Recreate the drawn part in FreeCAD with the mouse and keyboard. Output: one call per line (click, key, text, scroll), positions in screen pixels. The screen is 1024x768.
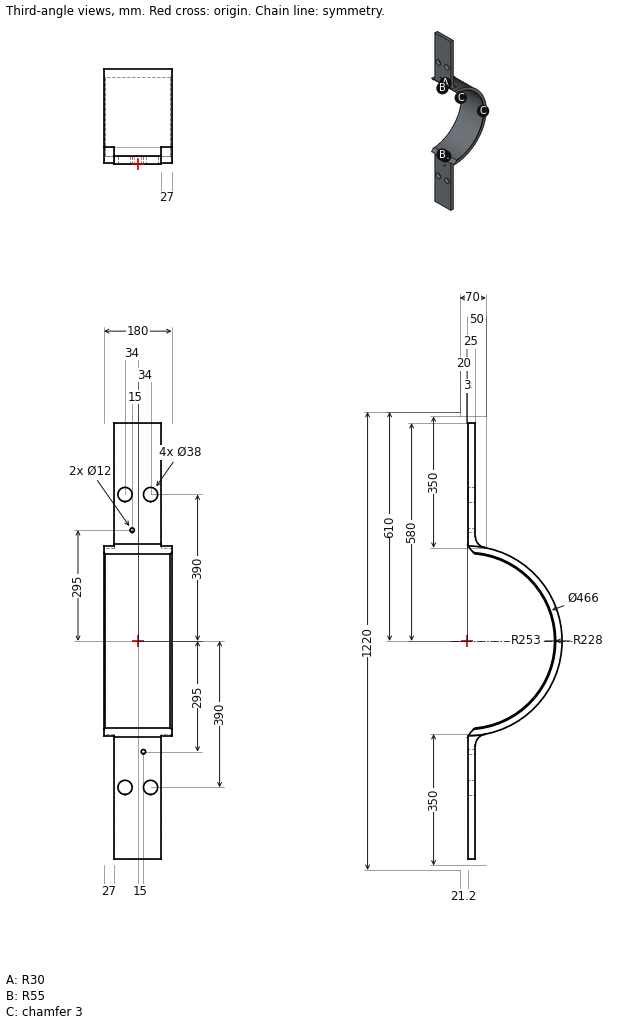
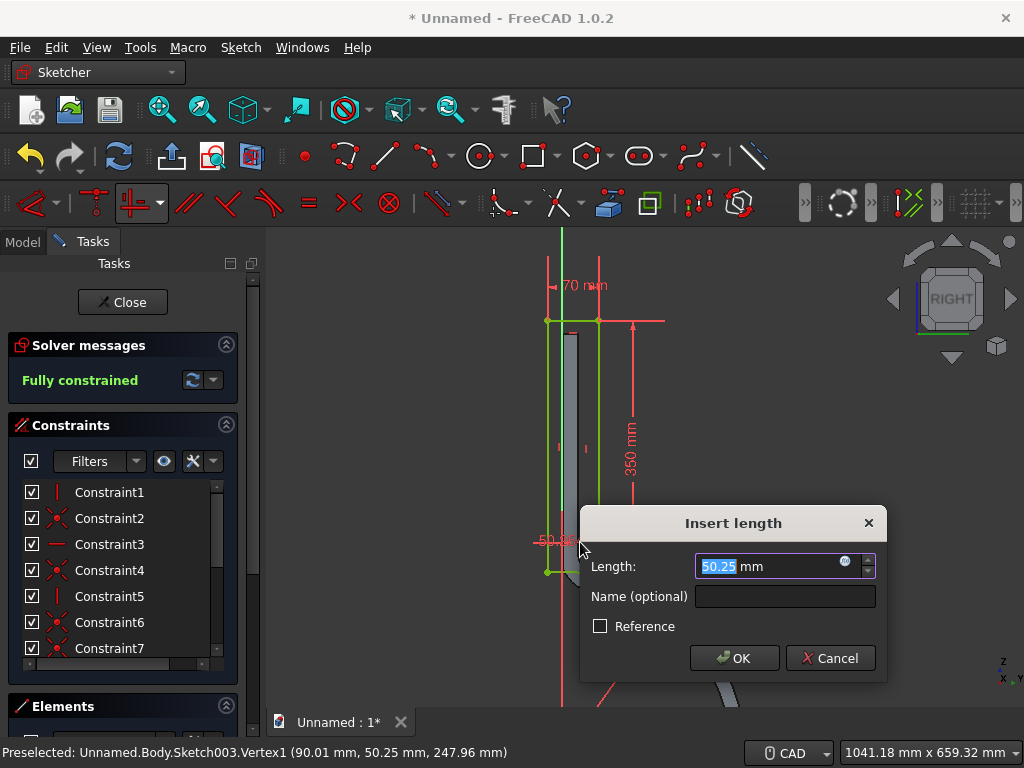
text(50)
key(Return)
key(Escape)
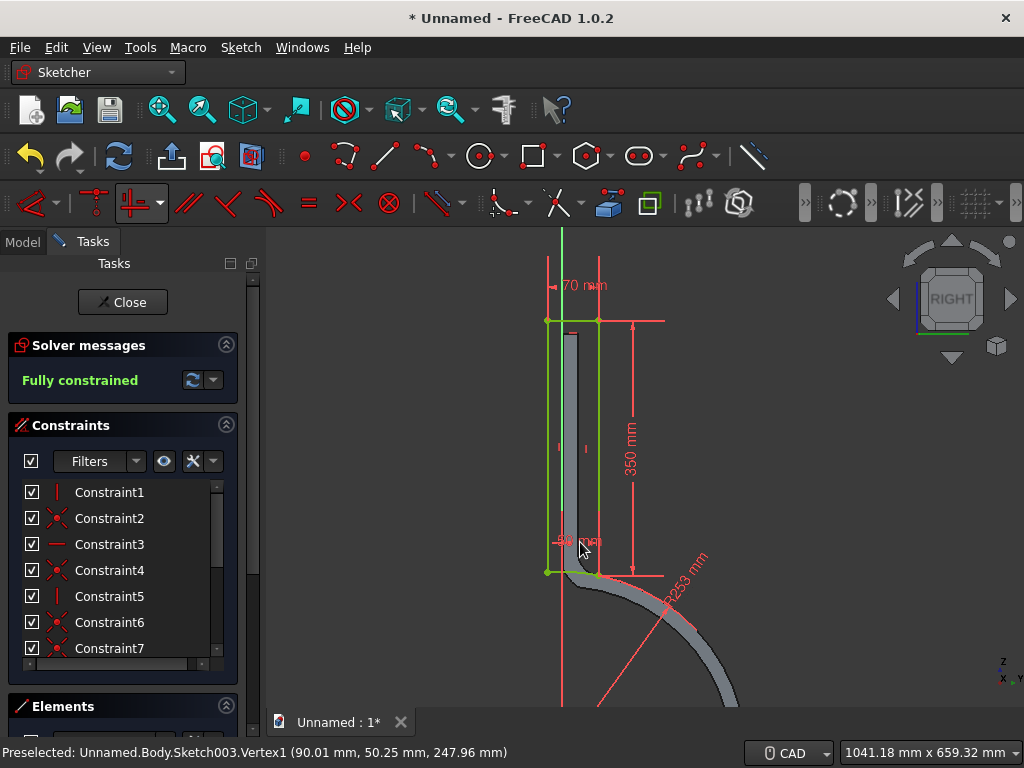
click(123, 302)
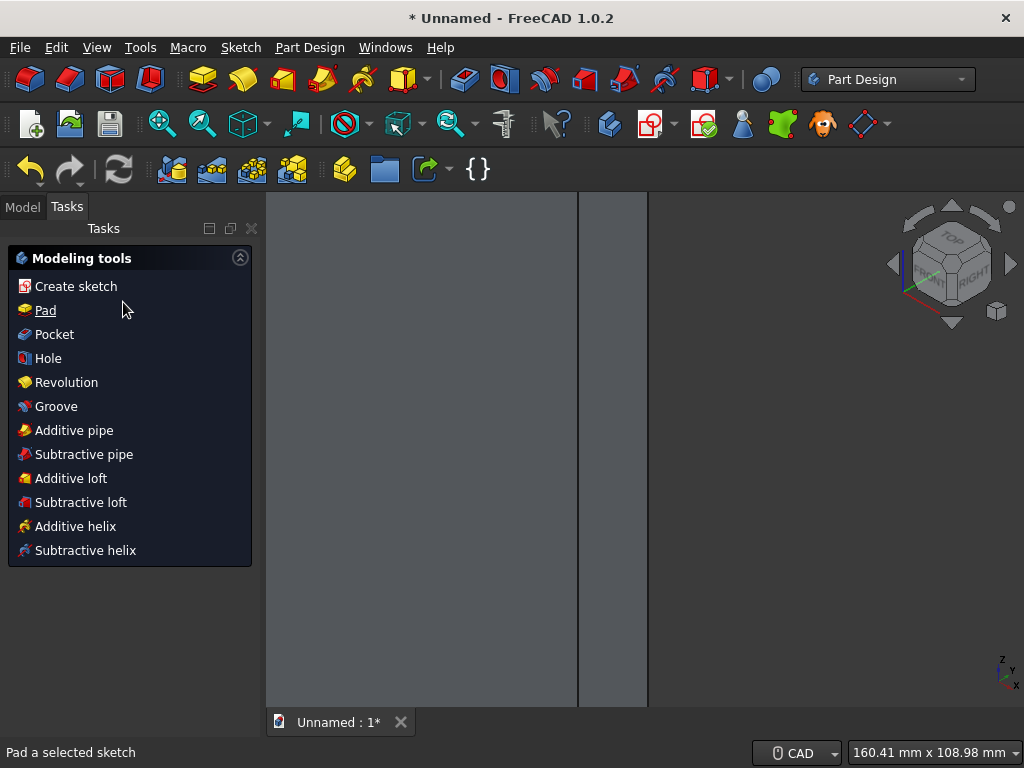
click(466, 80)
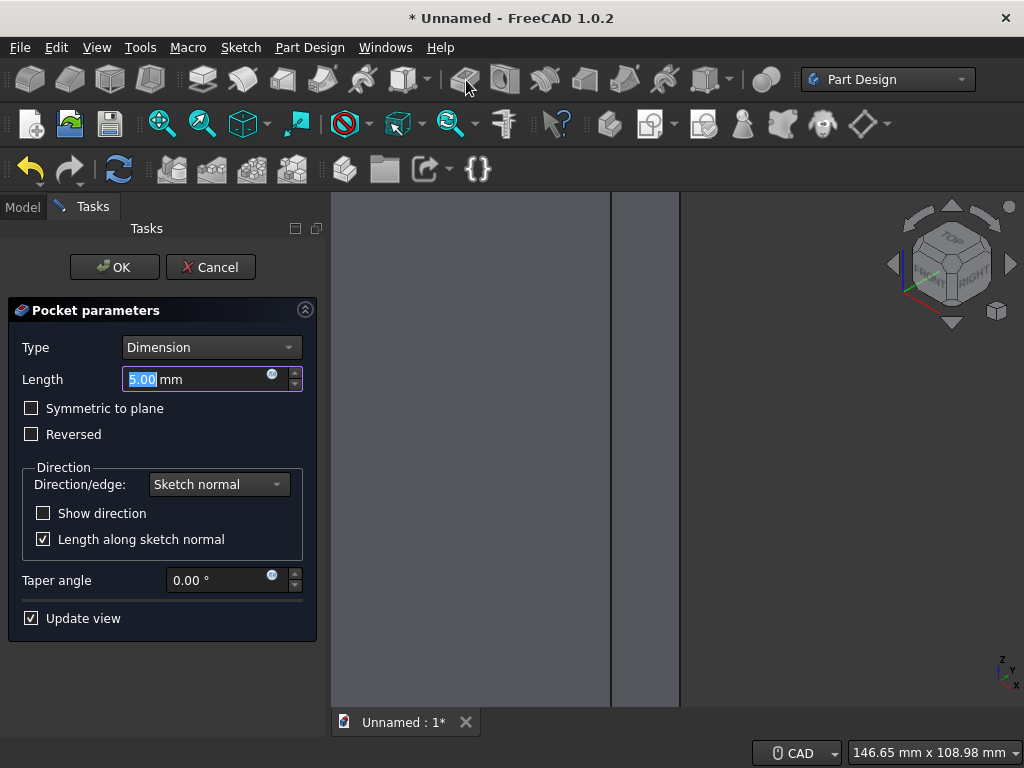
text(27)
key(Tab)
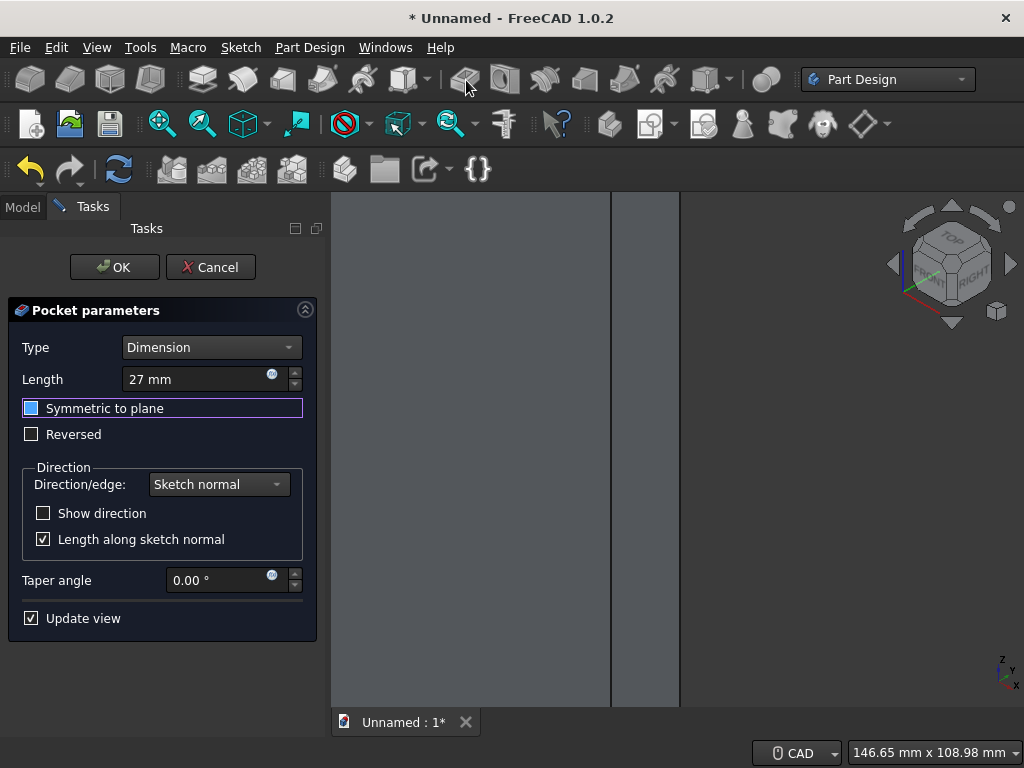
click(115, 267)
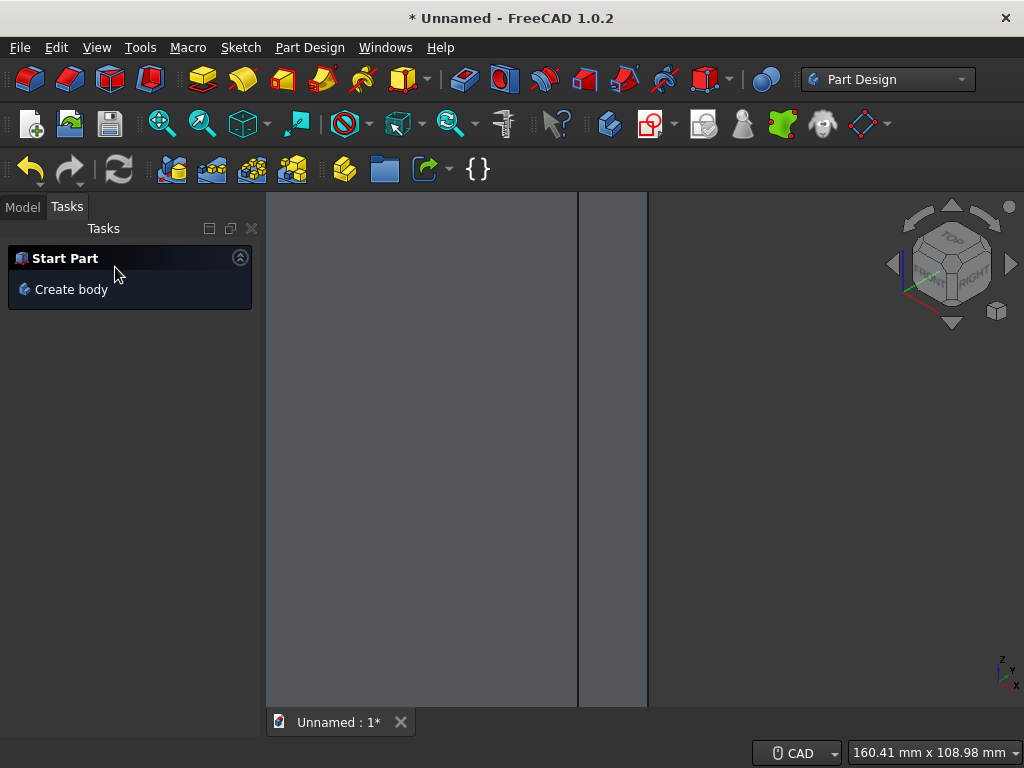
click(164, 124)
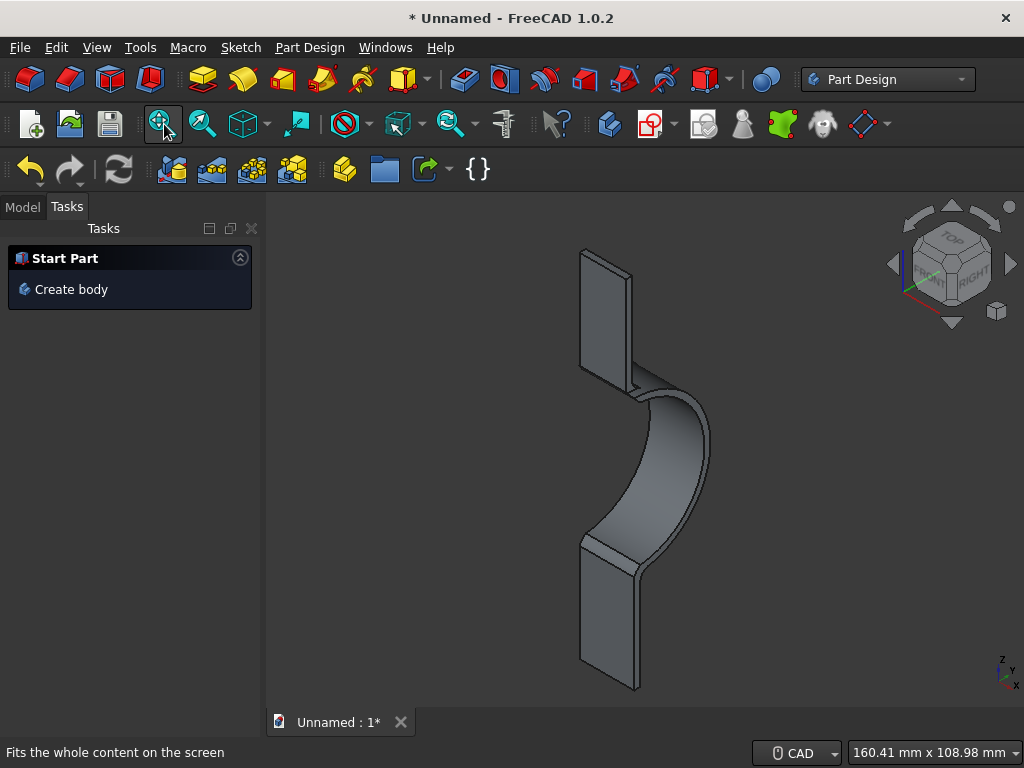
click(23, 206)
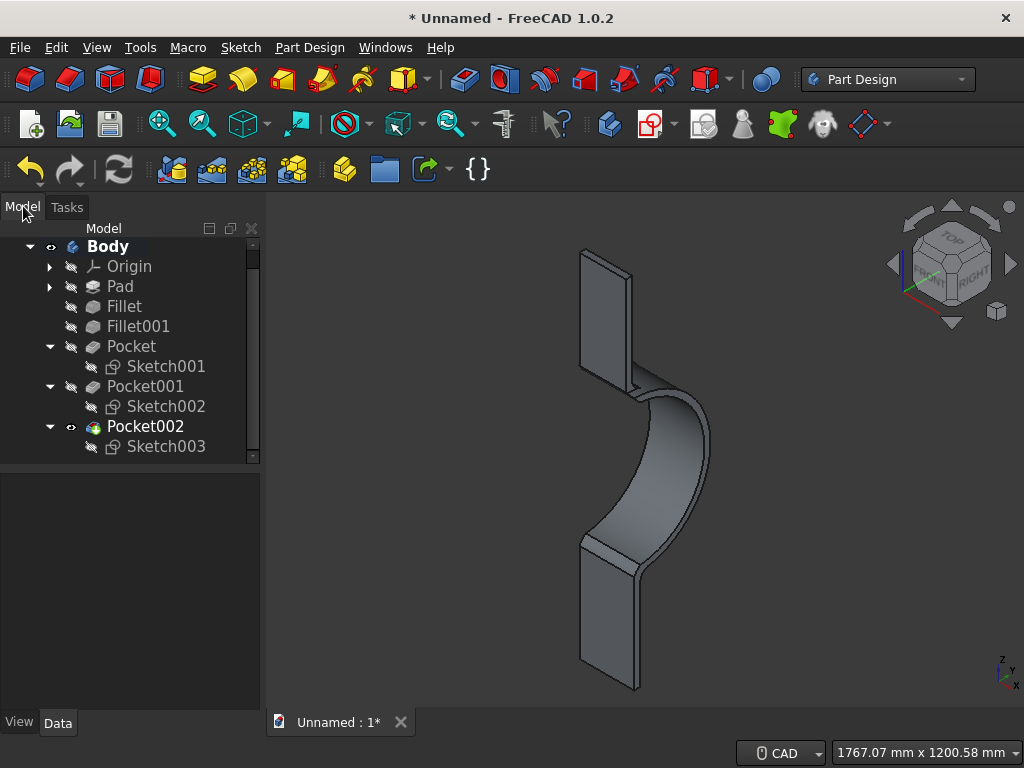
click(116, 427)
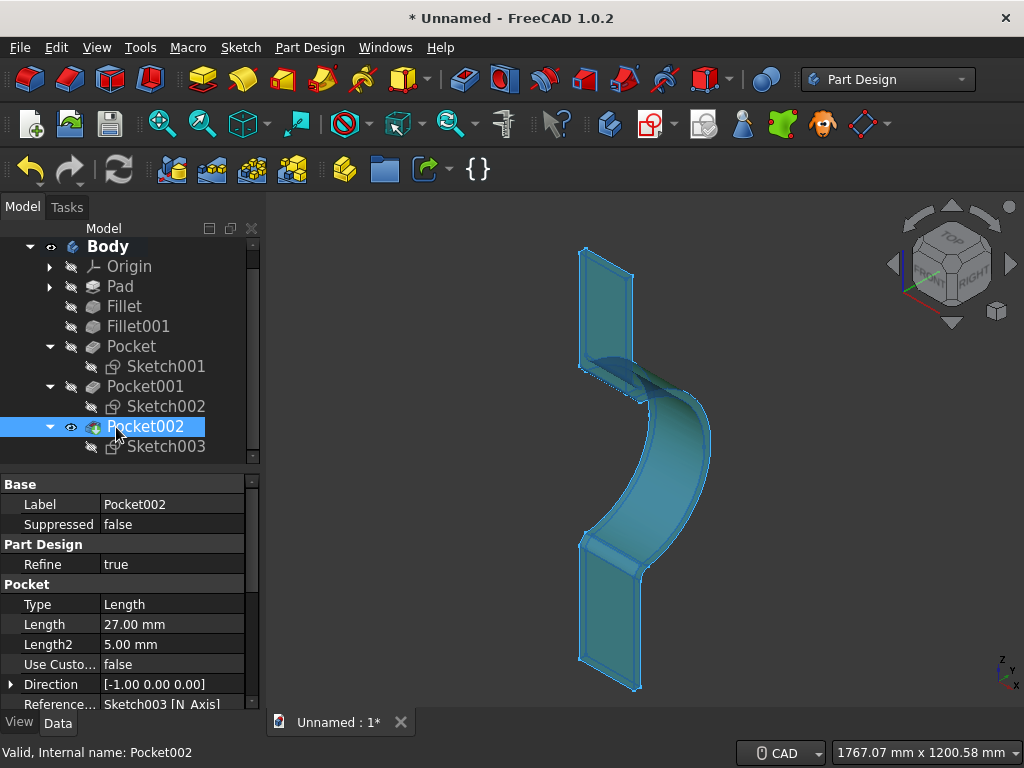
click(172, 170)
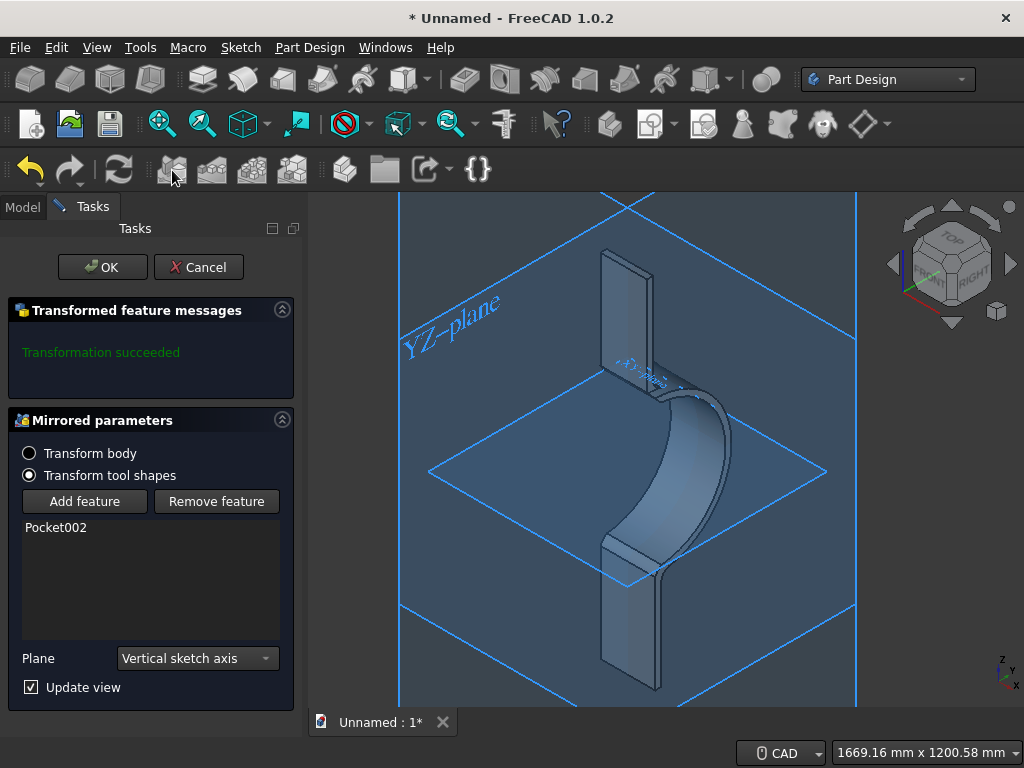
click(198, 658)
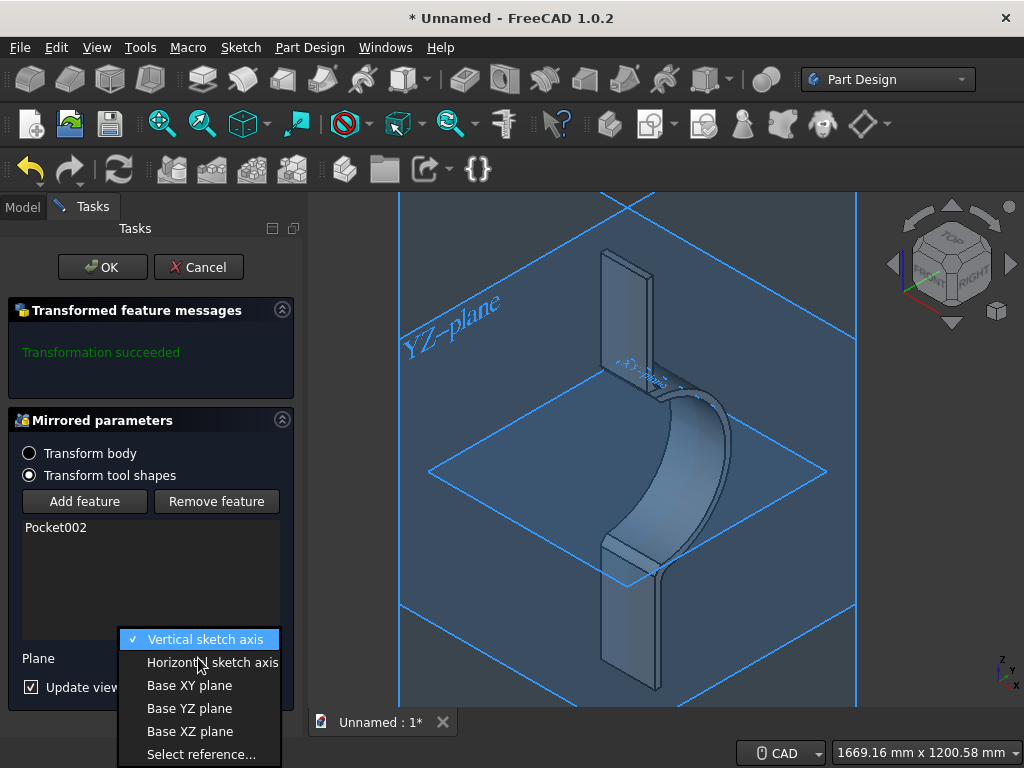
click(198, 686)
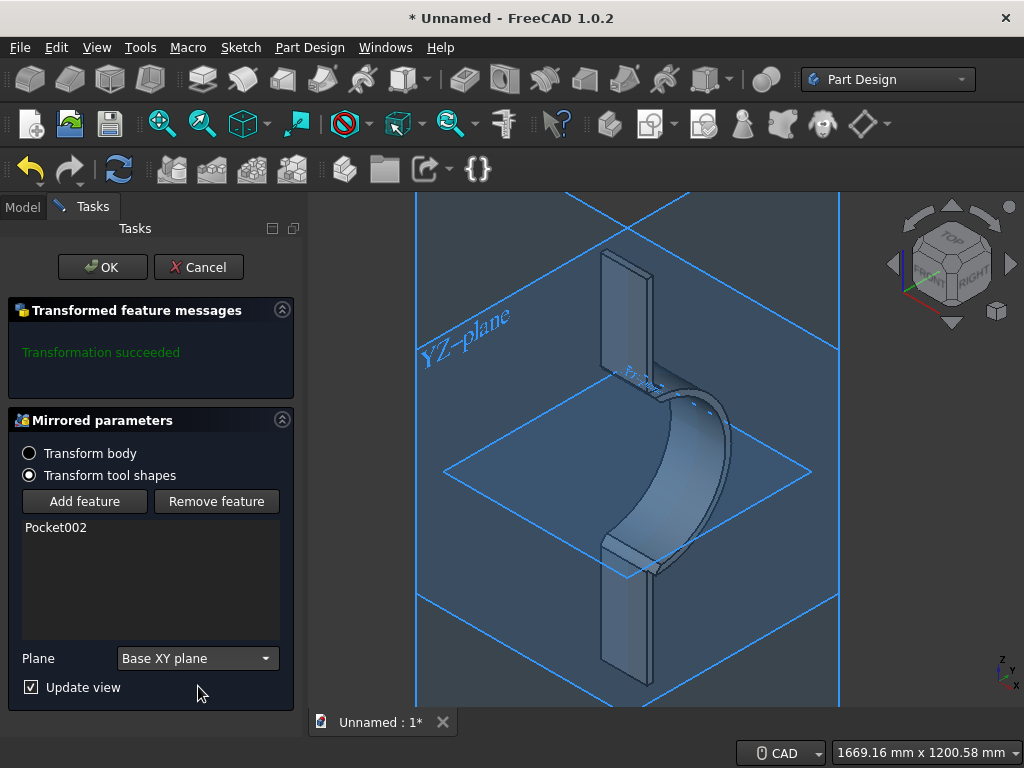
click(103, 267)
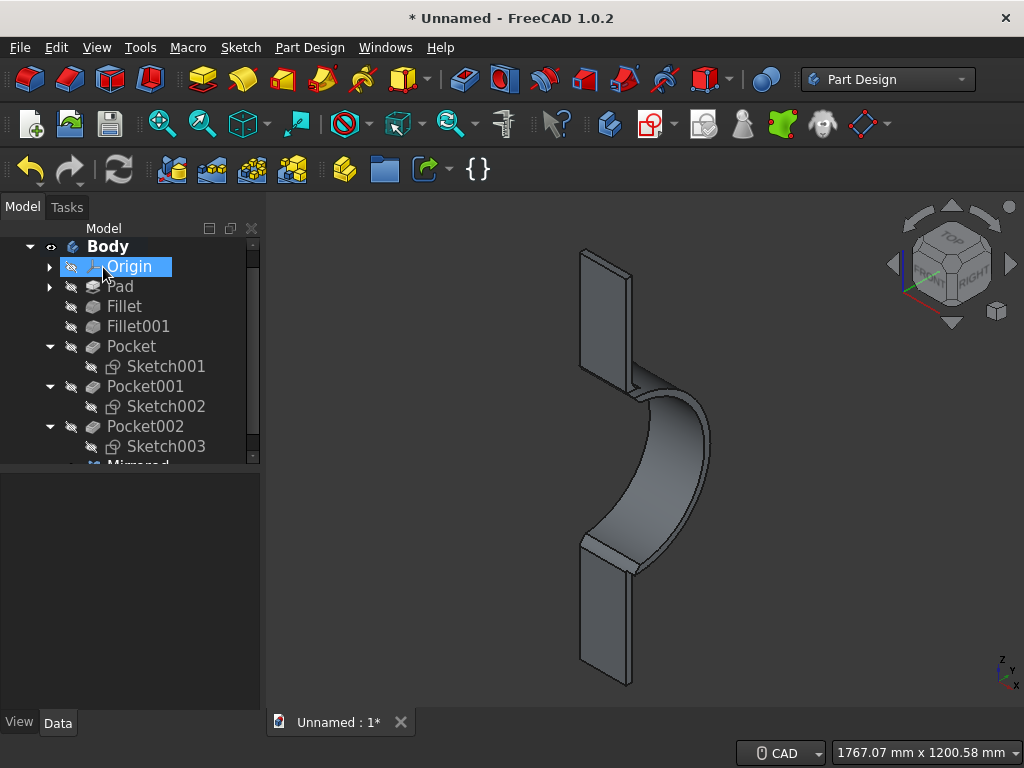
click(116, 427)